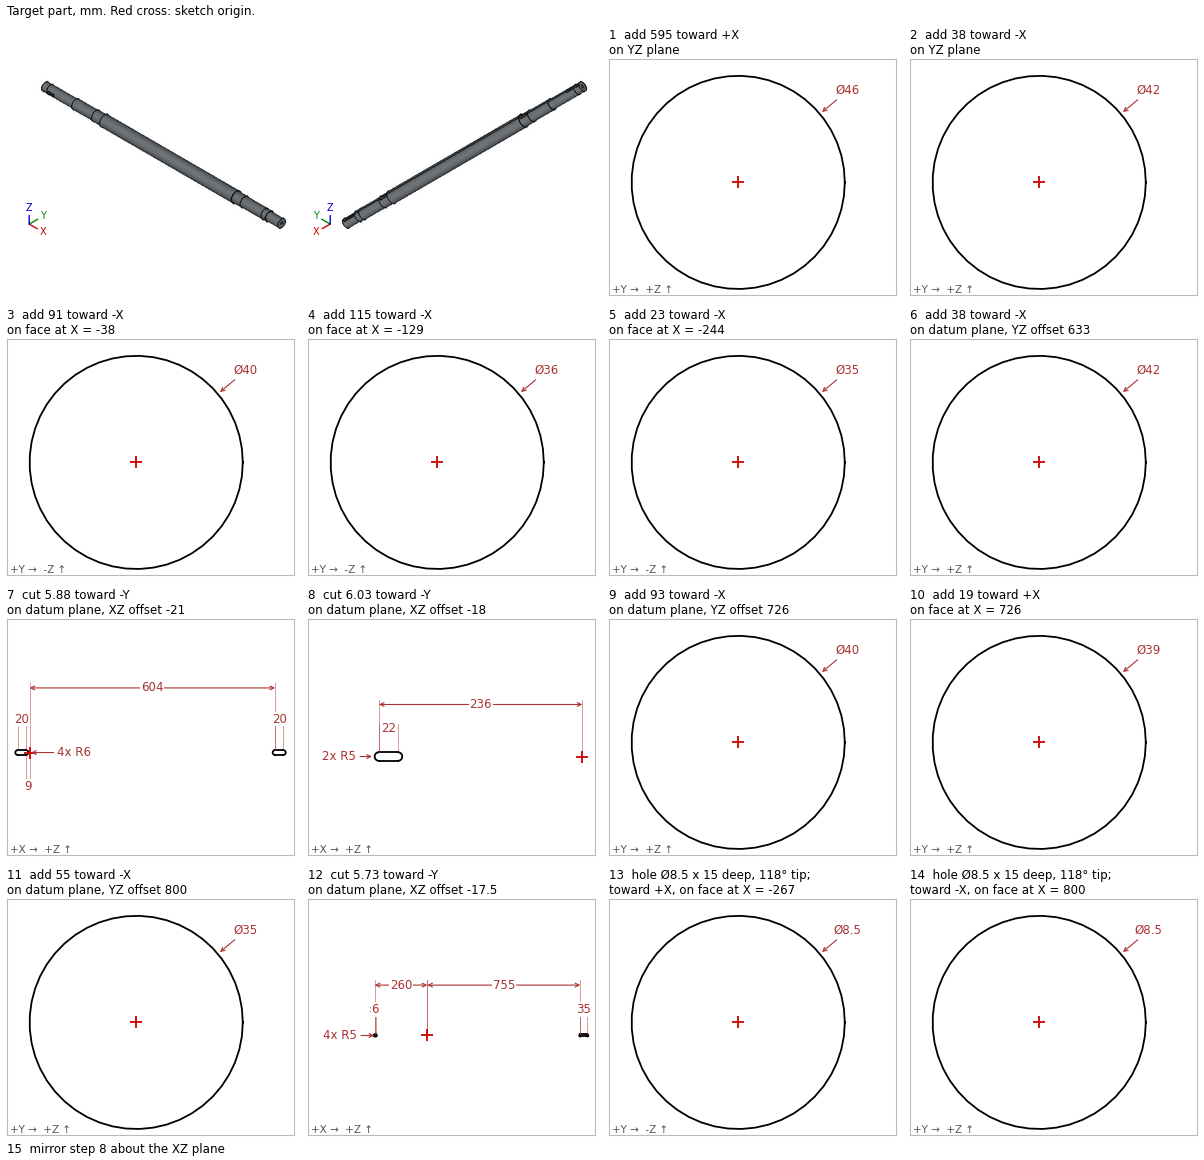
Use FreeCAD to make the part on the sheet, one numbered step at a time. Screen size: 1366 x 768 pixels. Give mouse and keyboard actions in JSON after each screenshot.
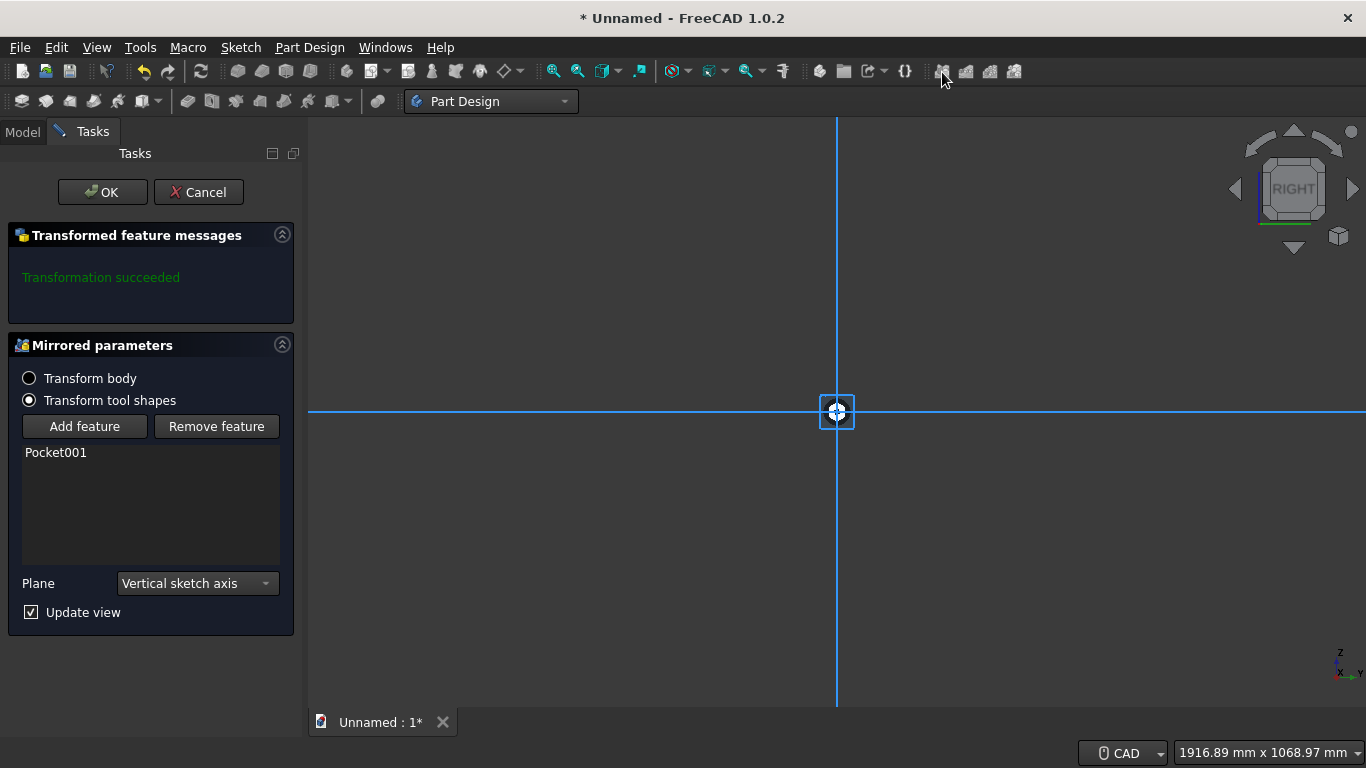
{"action": "left_click", "coordinate": [198, 584]}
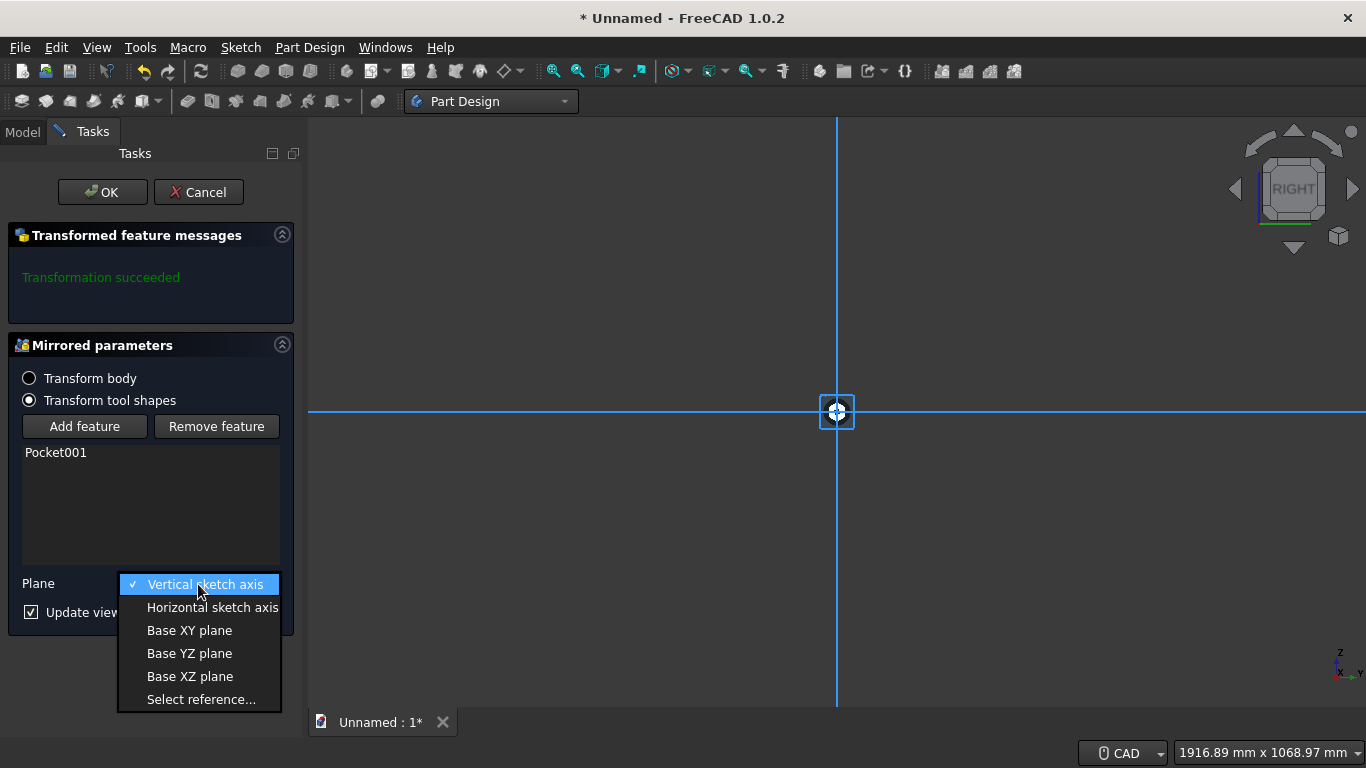
{"action": "left_click", "coordinate": [198, 676]}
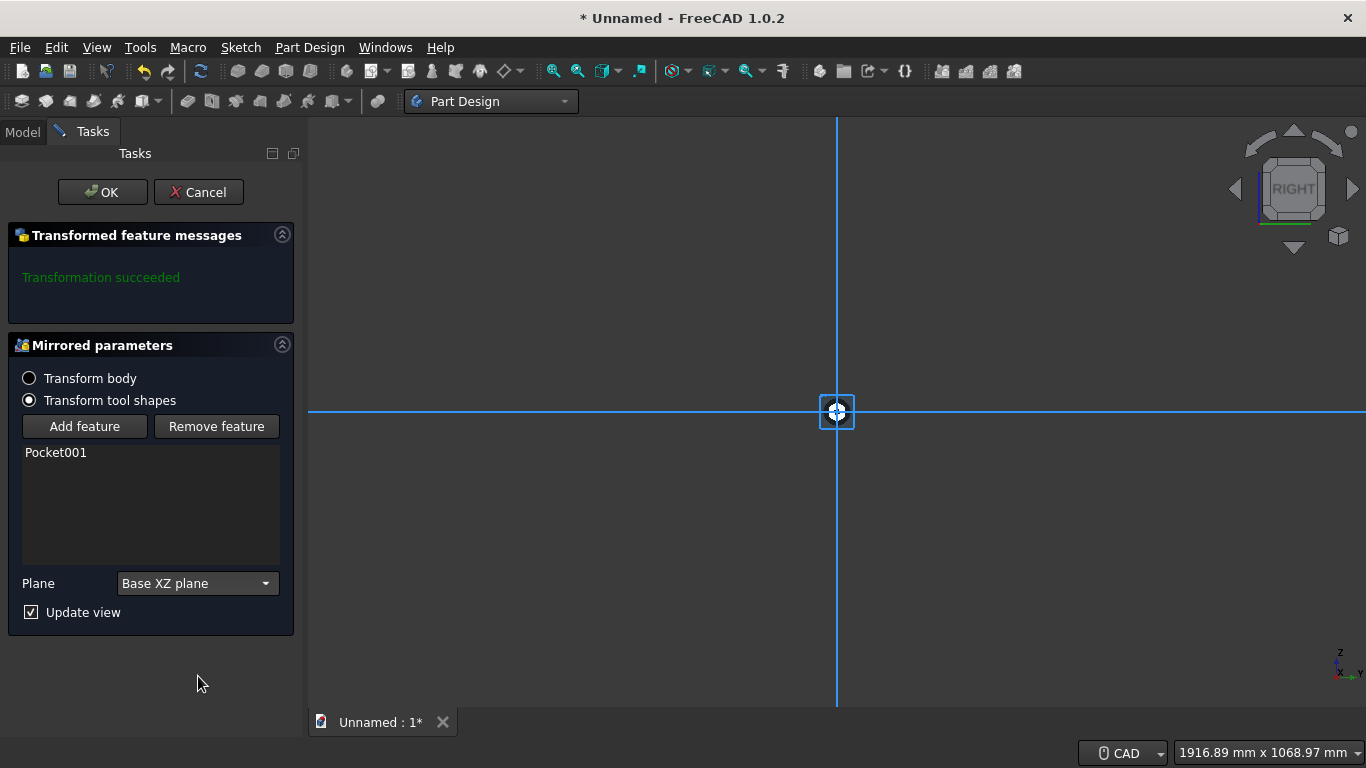
{"action": "left_click", "coordinate": [103, 192]}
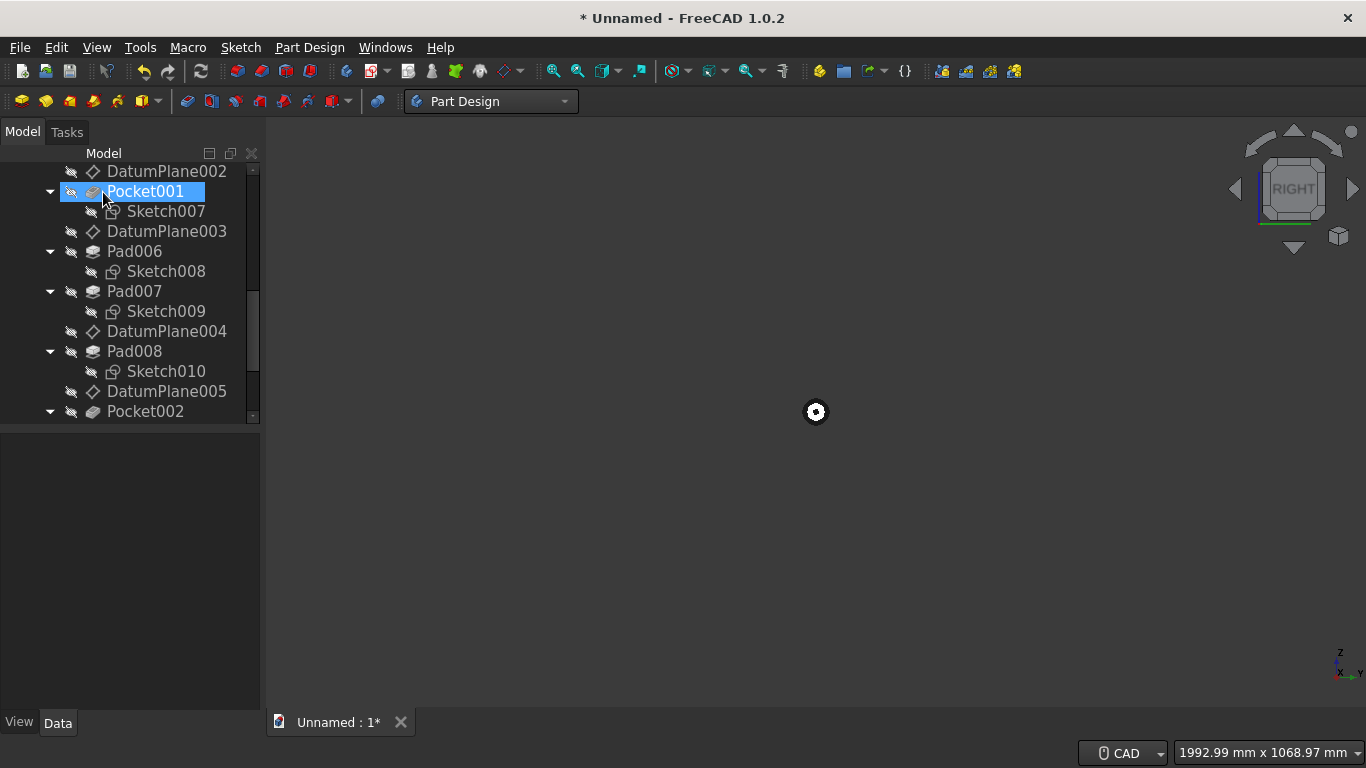
{"action": "key", "text": "0"}